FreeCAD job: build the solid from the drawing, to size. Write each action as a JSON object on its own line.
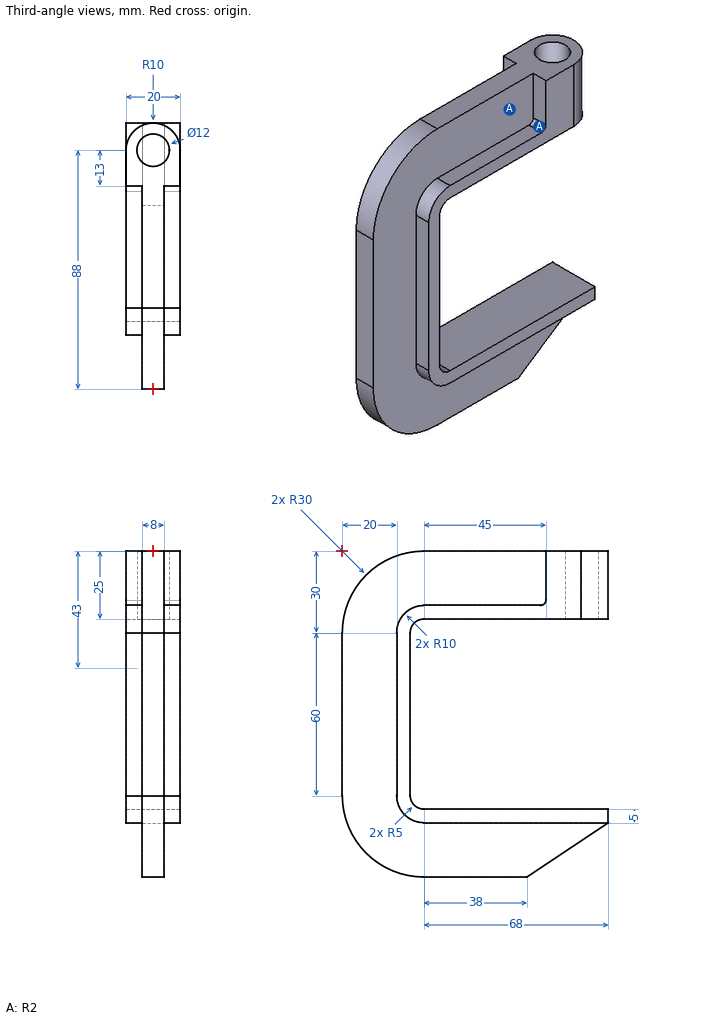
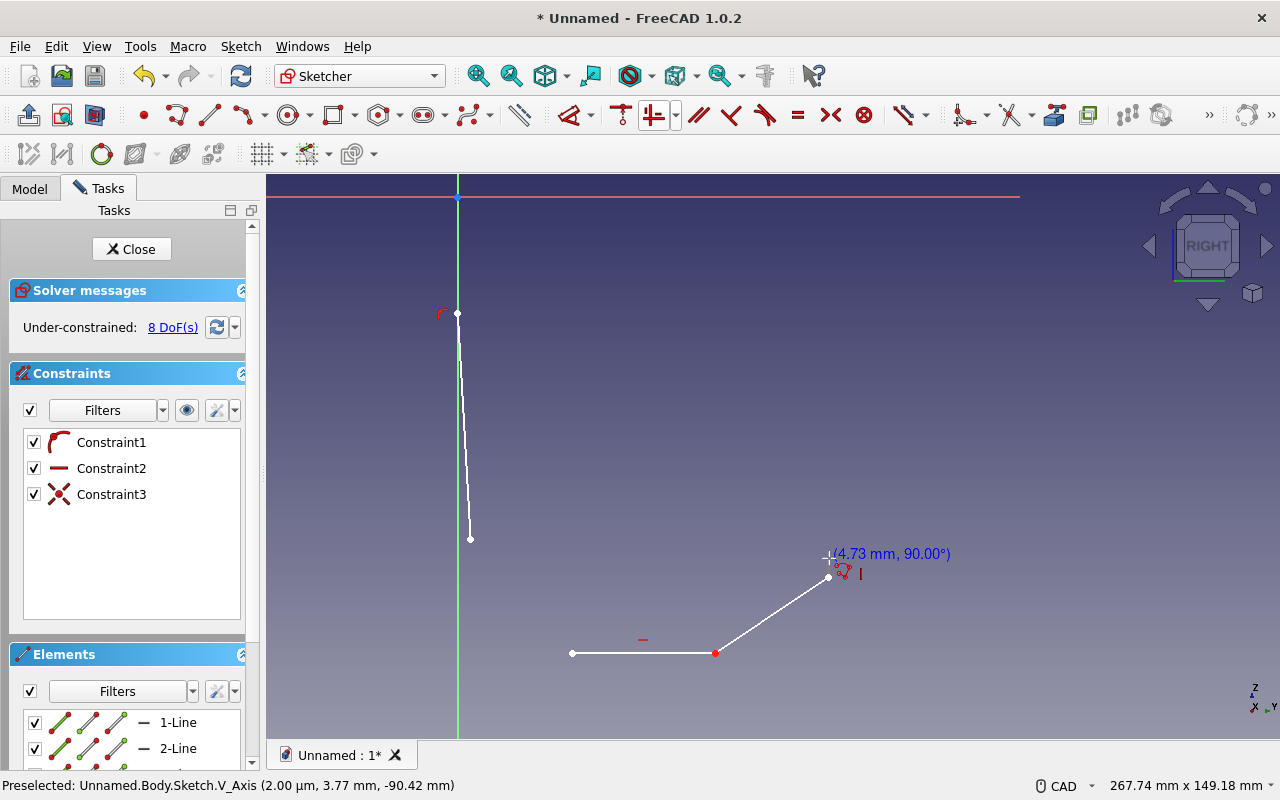
{"action": "left_click", "coordinate": [829, 557]}
{"action": "left_click", "coordinate": [571, 557]}
{"action": "right_click", "coordinate": [571, 557]}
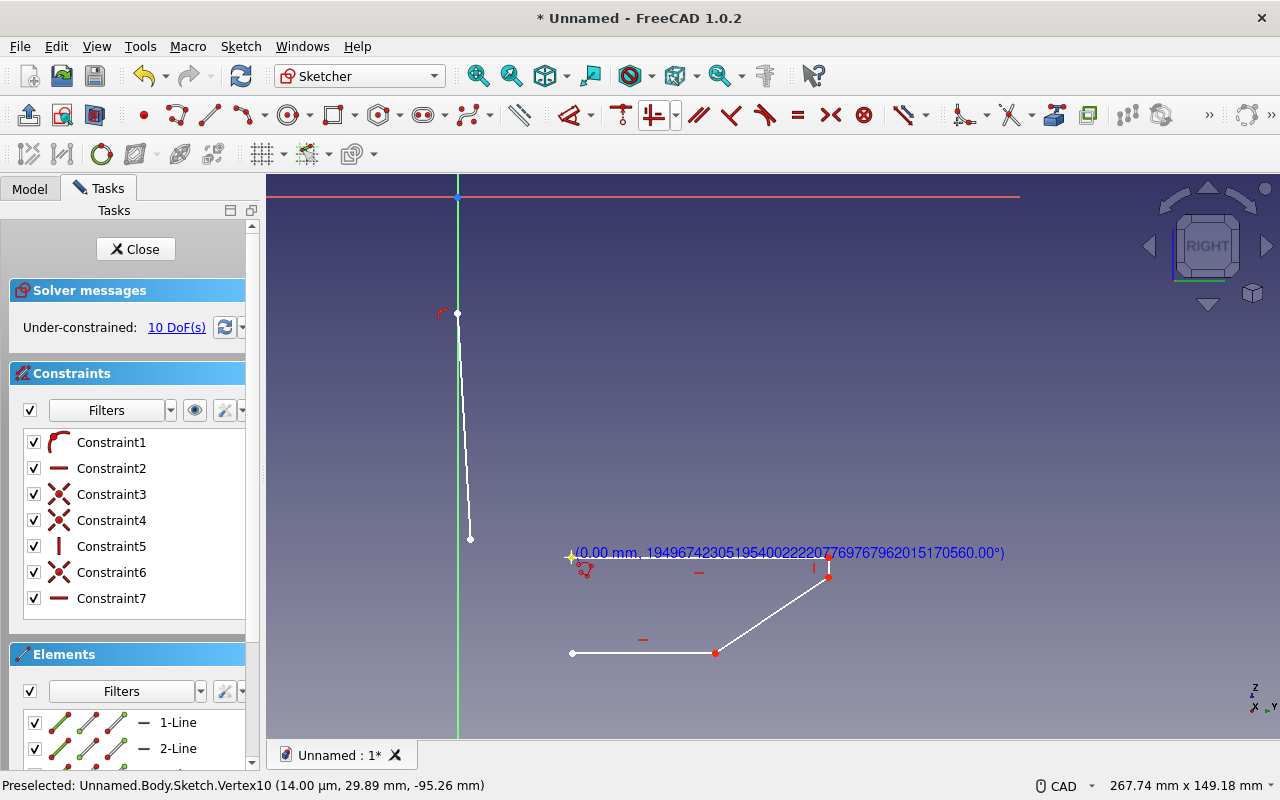
{"action": "left_click", "coordinate": [210, 116]}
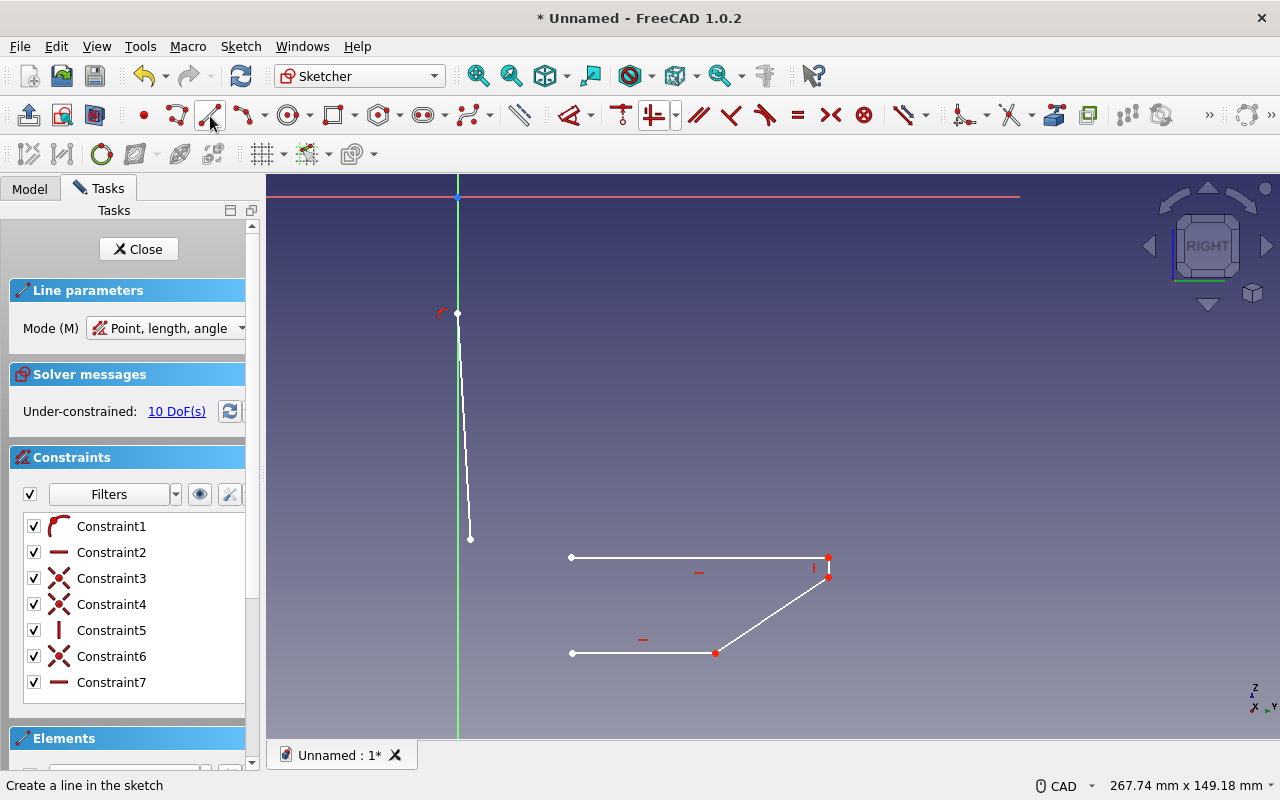
{"action": "left_click", "coordinate": [552, 538]}
{"action": "left_click", "coordinate": [552, 311]}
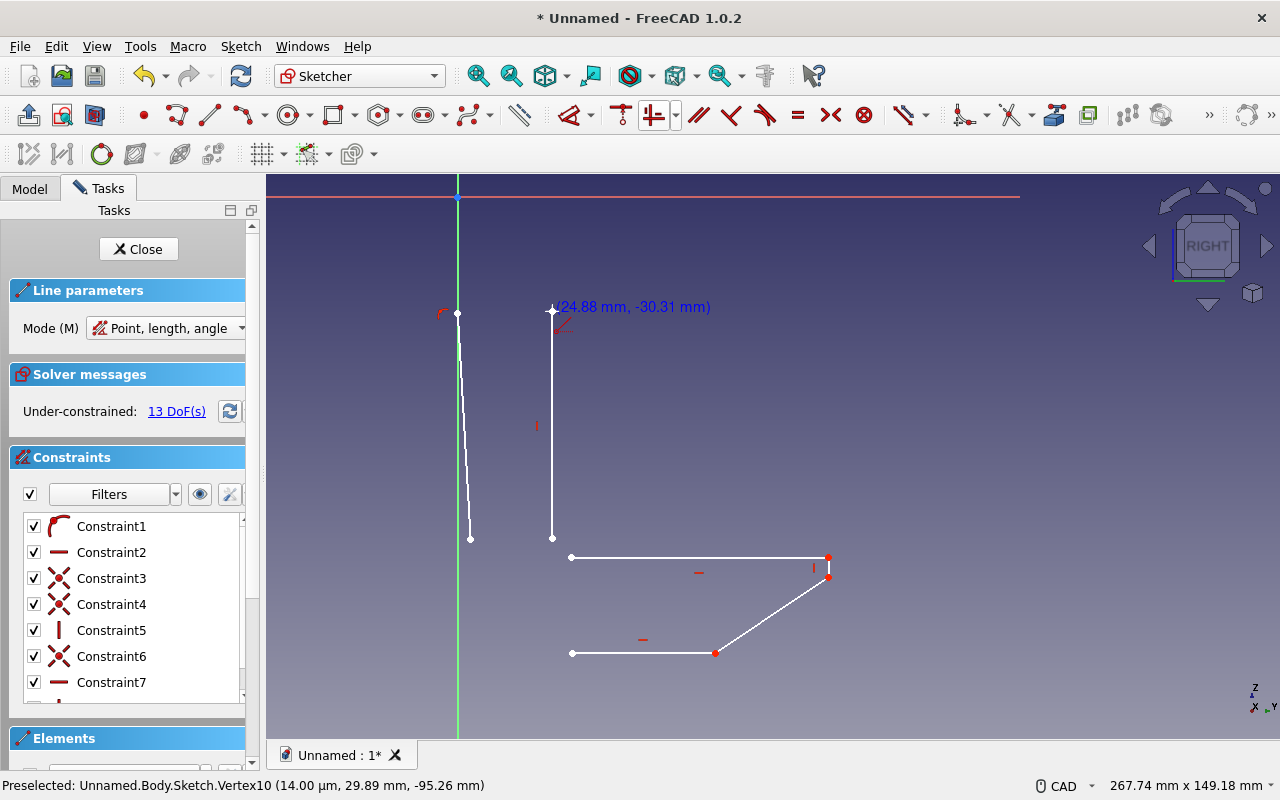
{"action": "key", "text": "g m"}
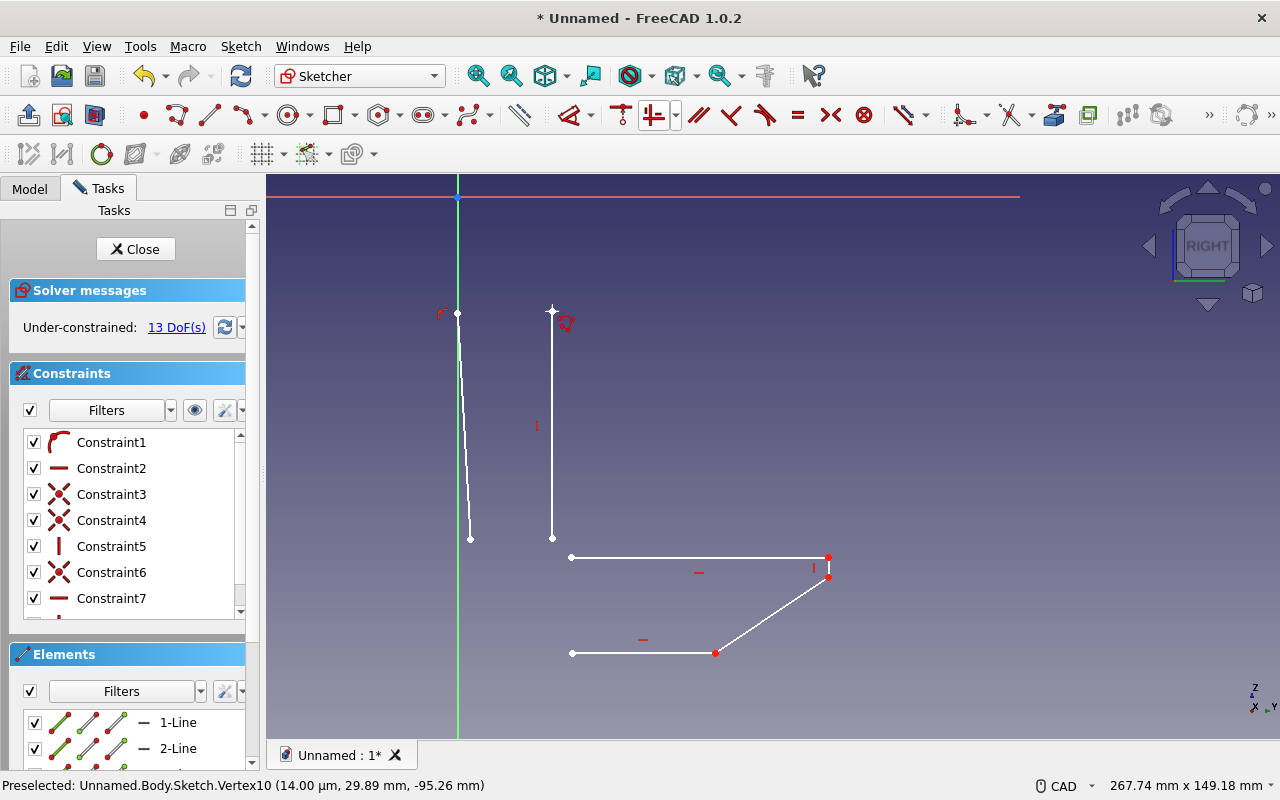
{"action": "left_click", "coordinate": [571, 292]}
{"action": "left_click", "coordinate": [742, 292]}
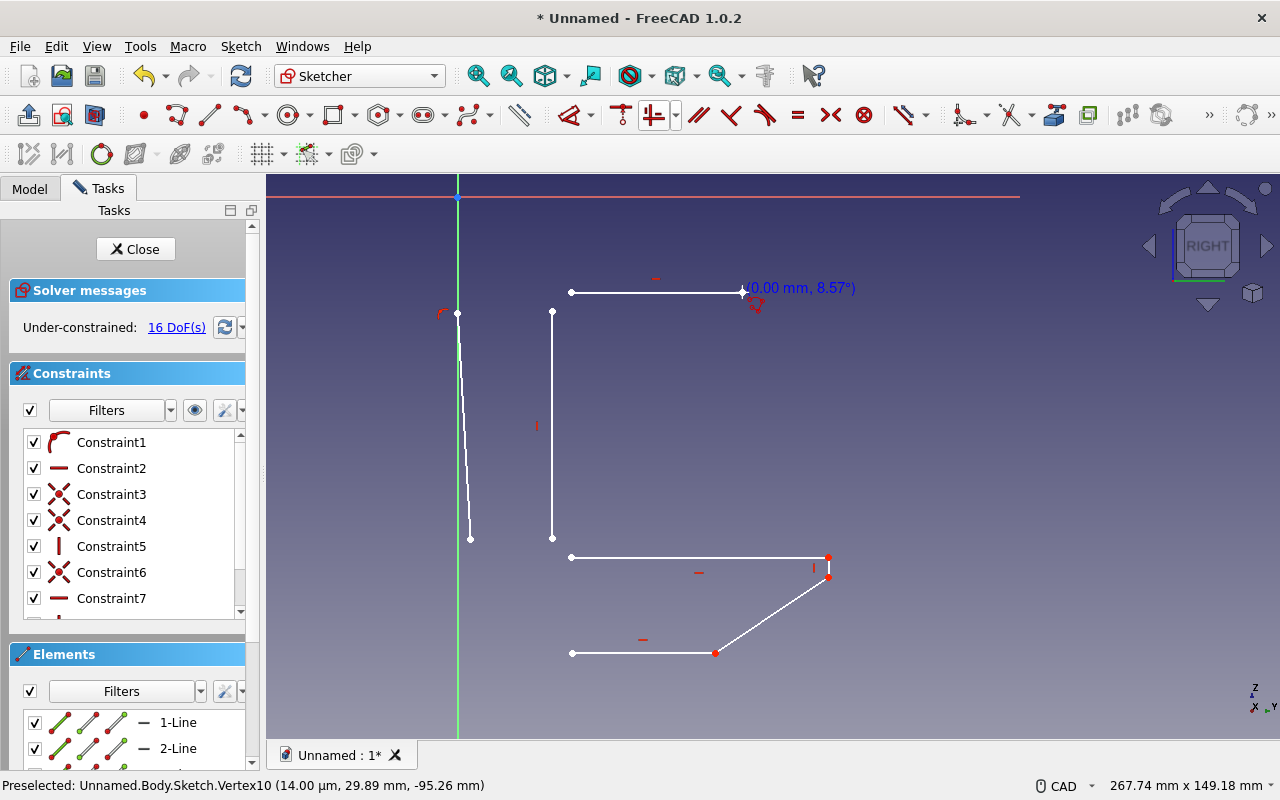
{"action": "scroll", "coordinate": [981, 601], "scroll_direction": "down", "scroll_amount": 1}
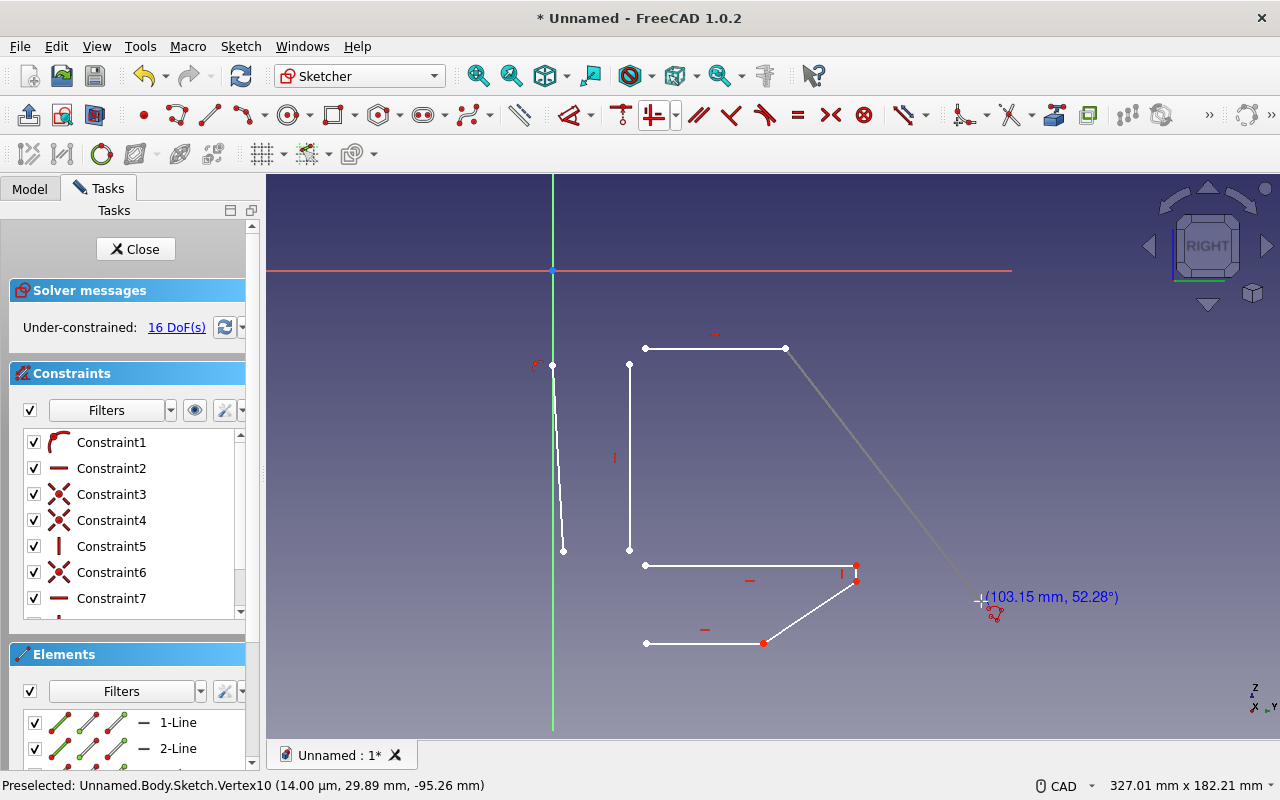
{"action": "left_click", "coordinate": [785, 271]}
{"action": "left_click", "coordinate": [646, 280]}
{"action": "right_click", "coordinate": [646, 280]}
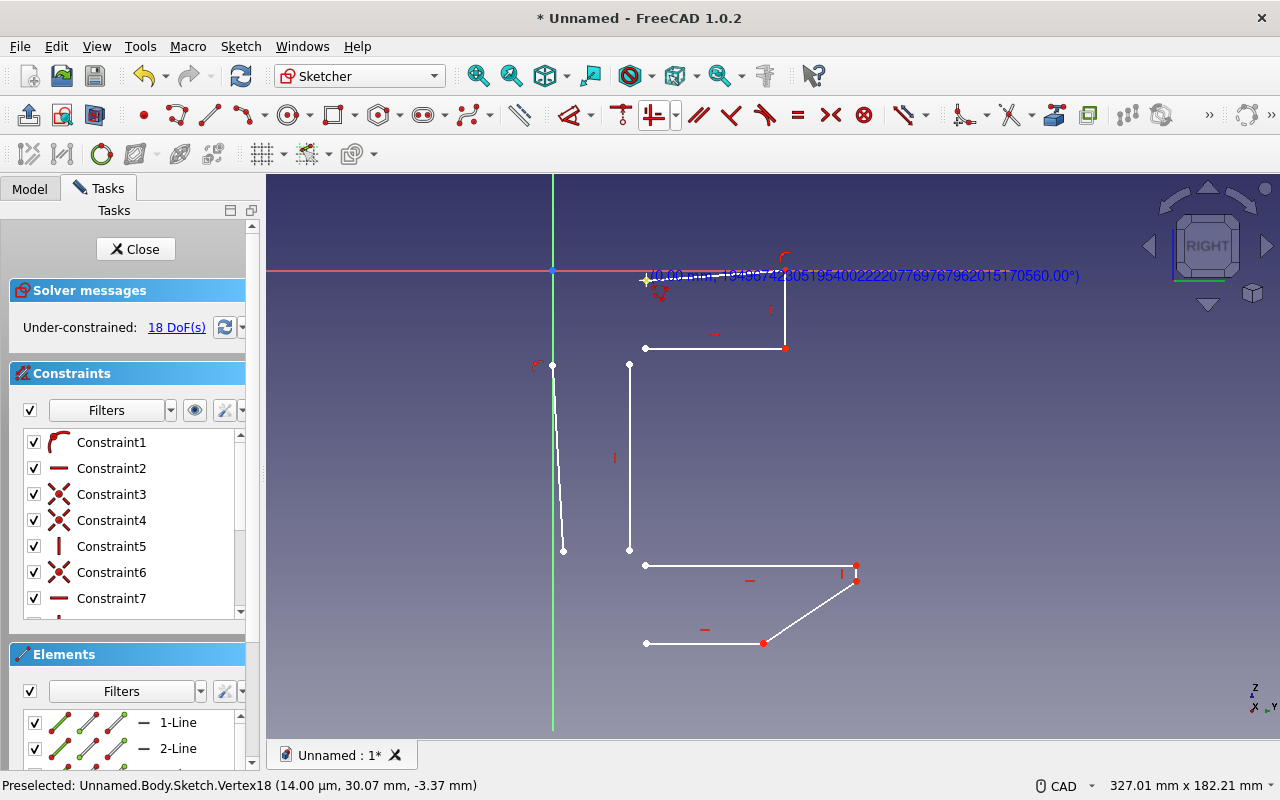
{"action": "key", "text": "g 3 a"}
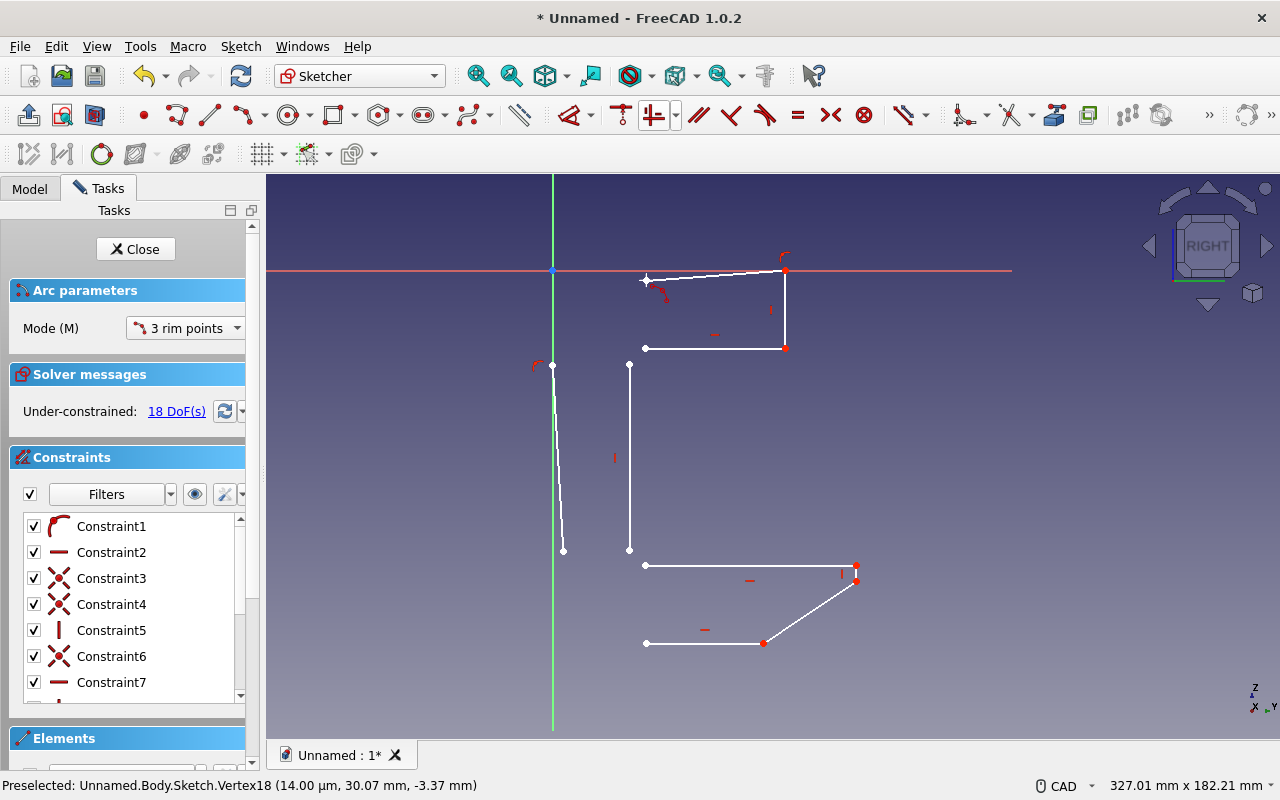
{"action": "left_click", "coordinate": [563, 551]}
{"action": "left_click", "coordinate": [646, 644]}
{"action": "left_click", "coordinate": [580, 615]}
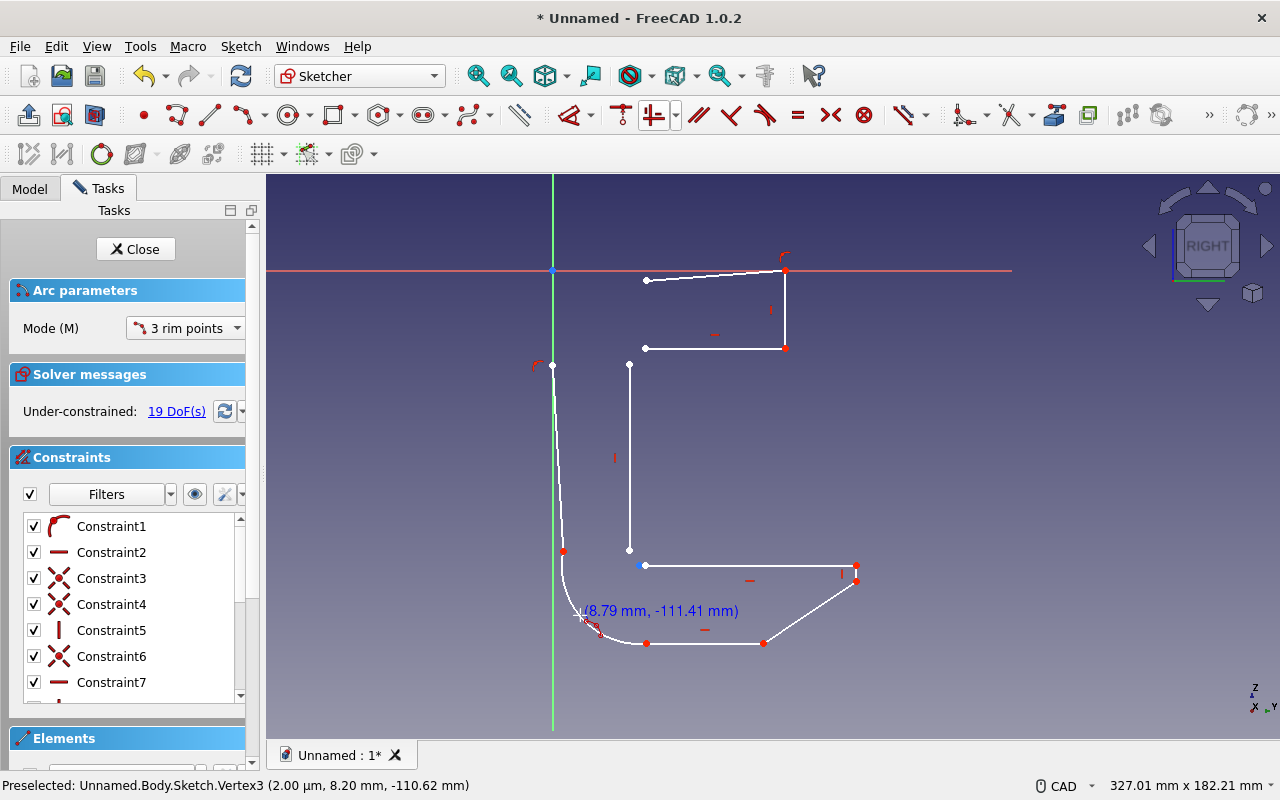
{"action": "left_click", "coordinate": [645, 566]}
{"action": "left_click", "coordinate": [630, 550]}